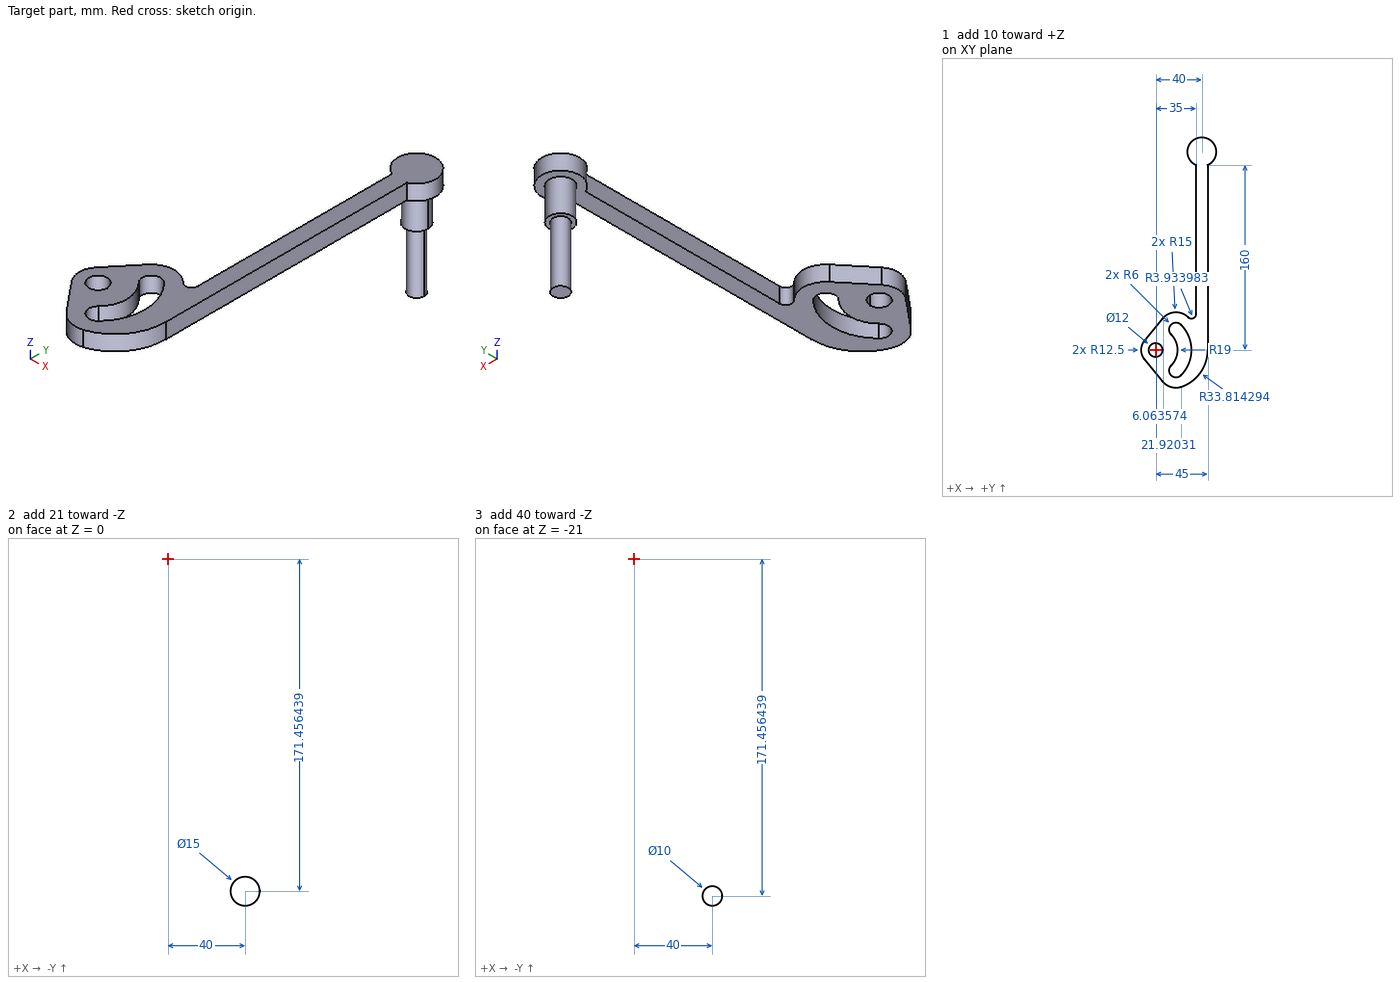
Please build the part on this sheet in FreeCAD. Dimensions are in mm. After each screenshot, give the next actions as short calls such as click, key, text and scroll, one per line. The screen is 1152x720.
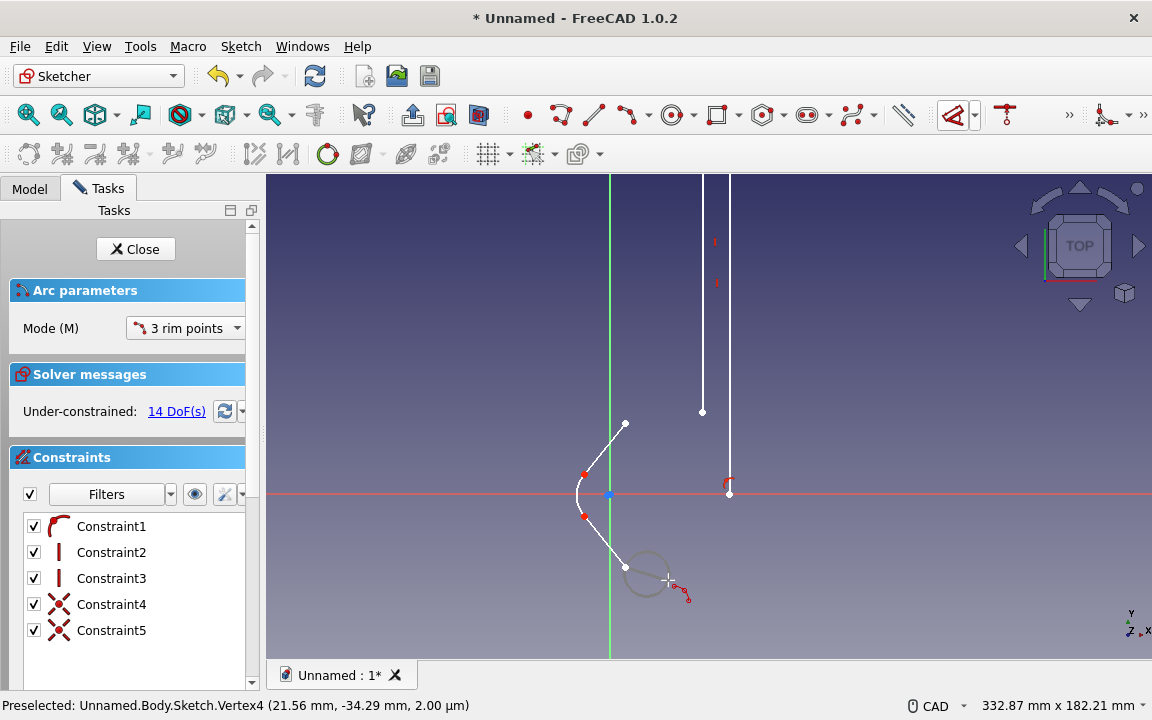
scroll(645, 580, up, 5)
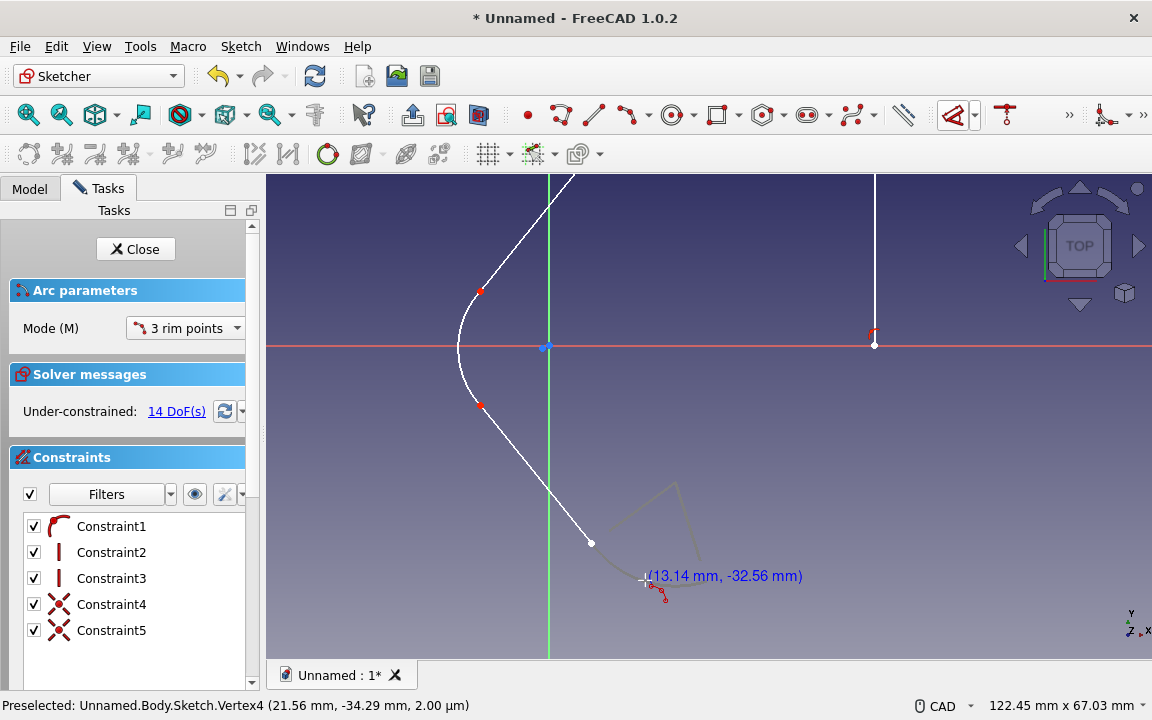
click(645, 577)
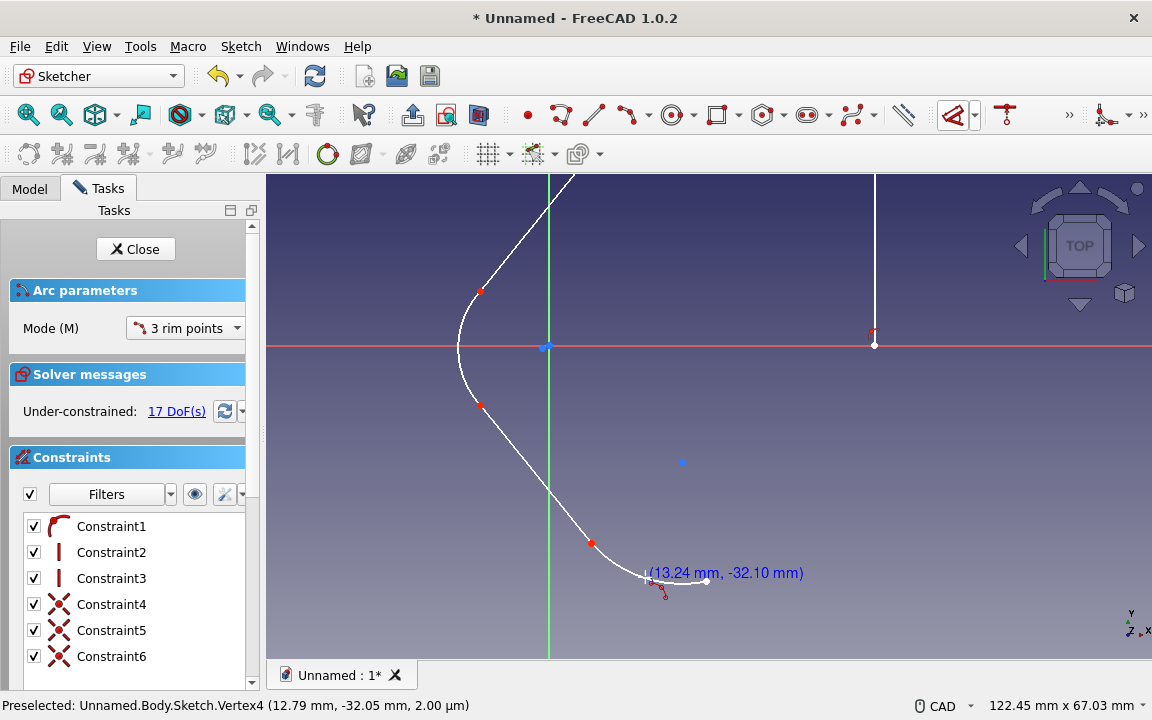
scroll(634, 573, down, 8)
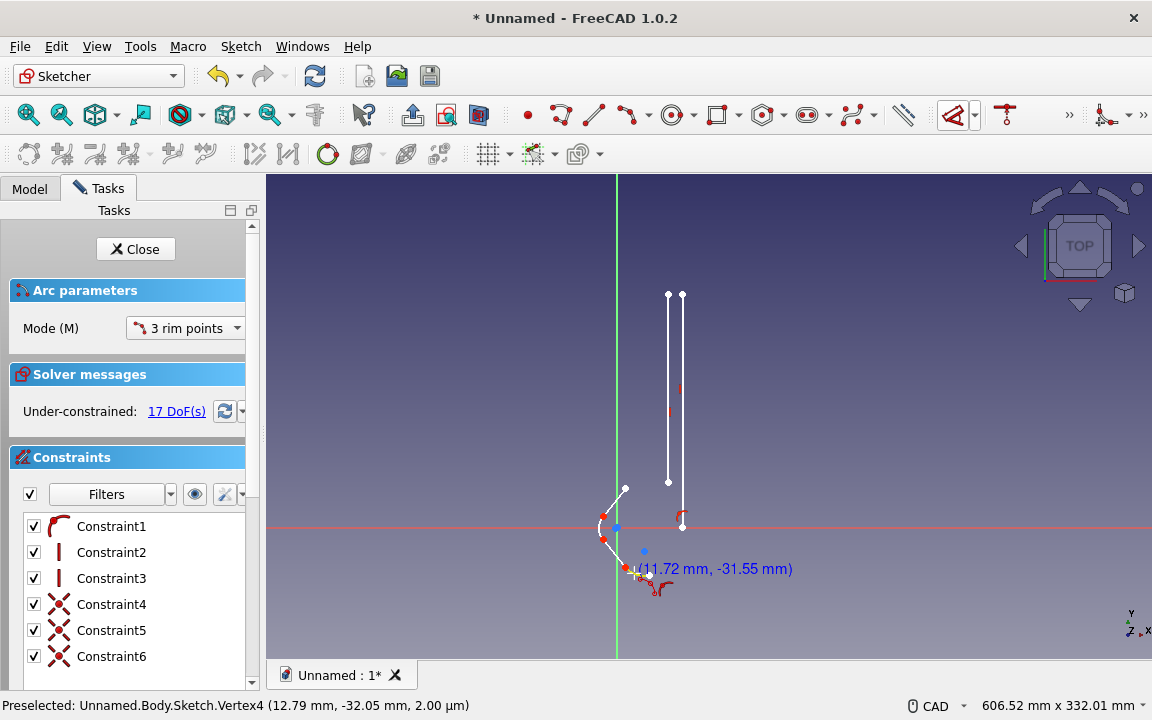
click(649, 575)
click(683, 528)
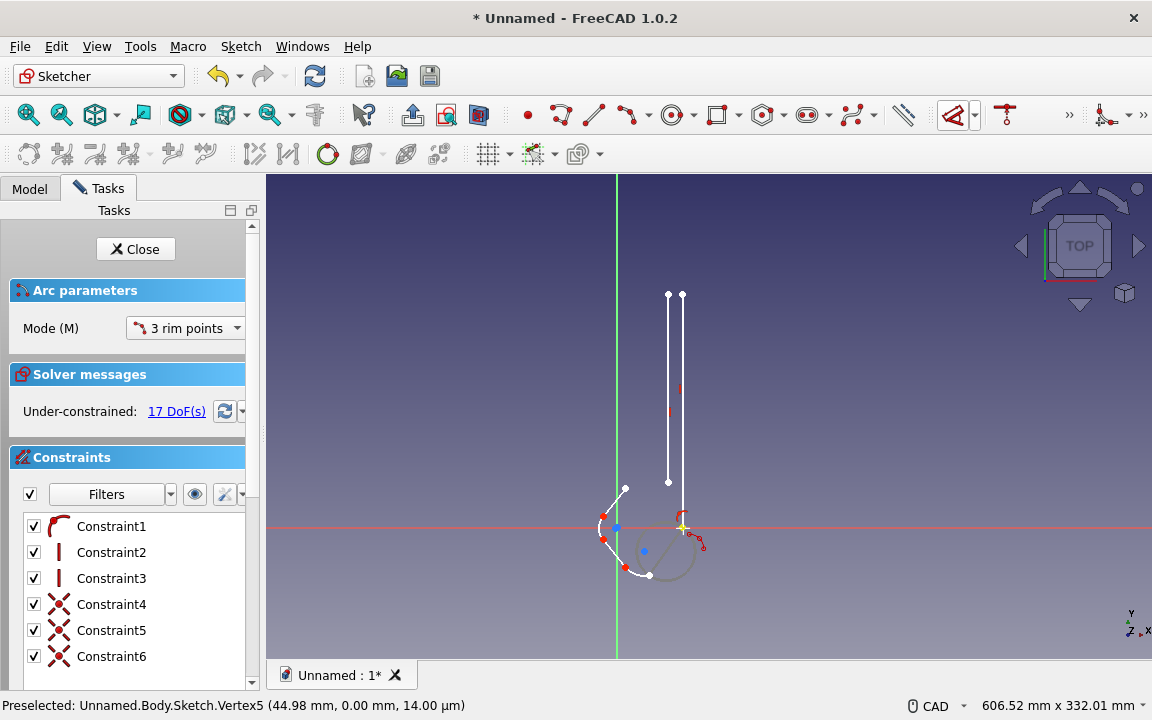
scroll(674, 557, up, 3)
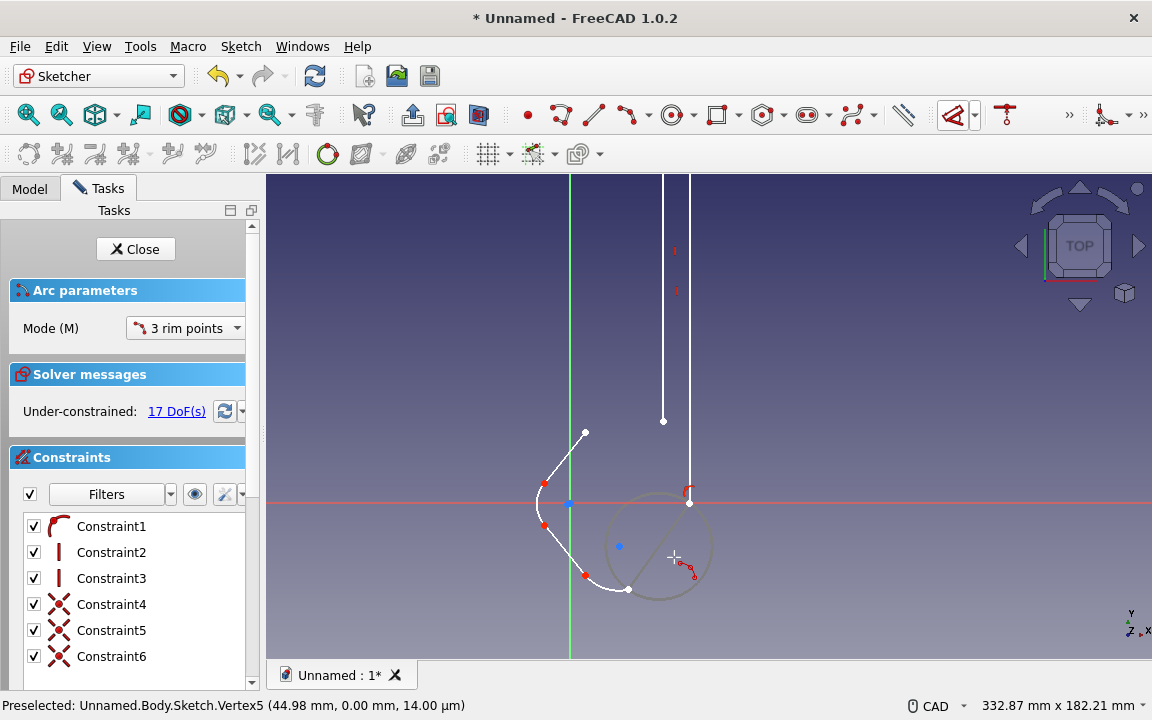
click(673, 556)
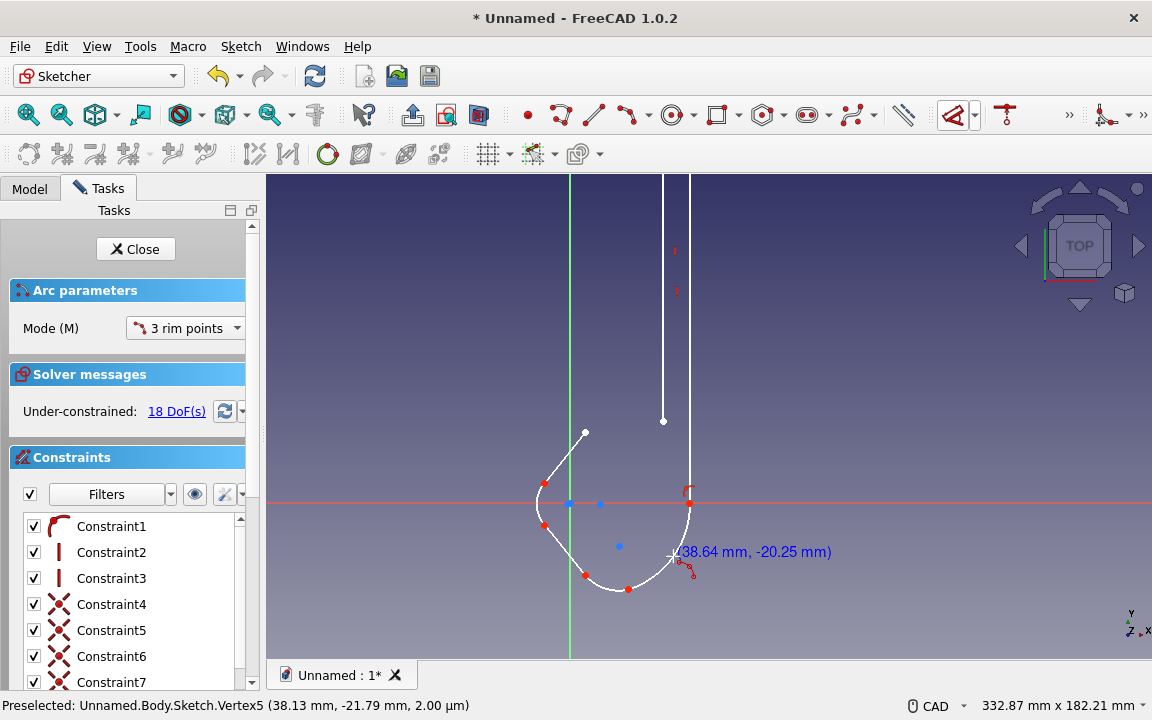
scroll(673, 557, down, 3)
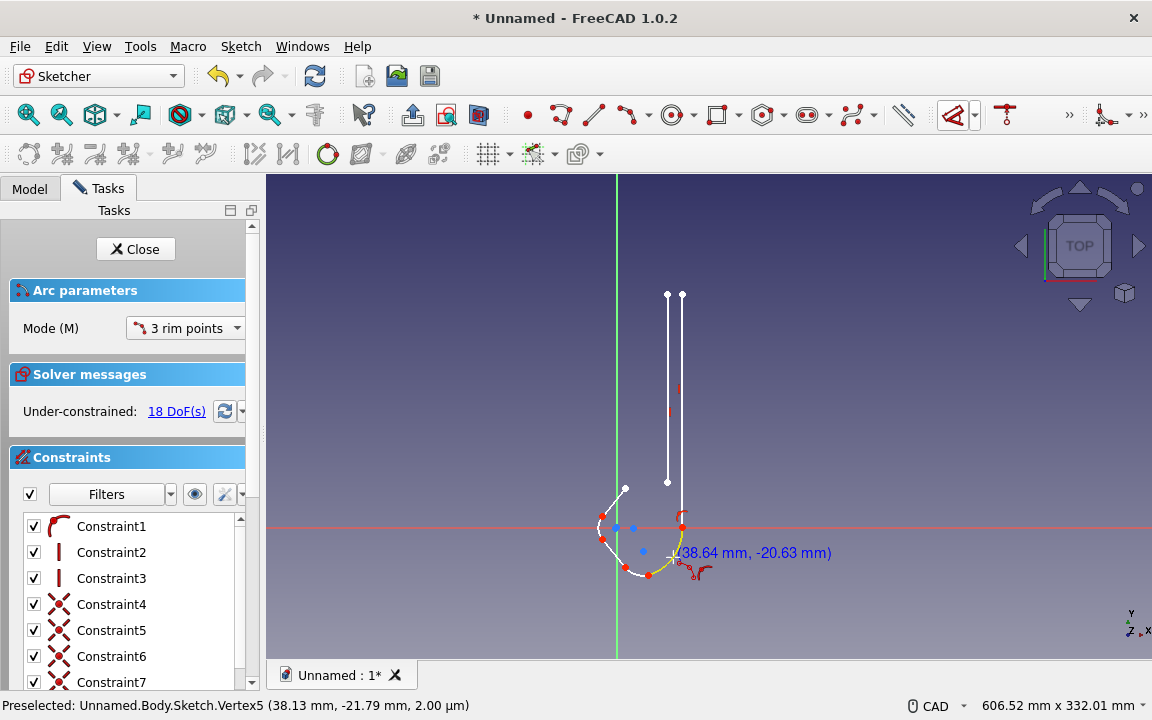
click(682, 295)
click(668, 295)
click(675, 259)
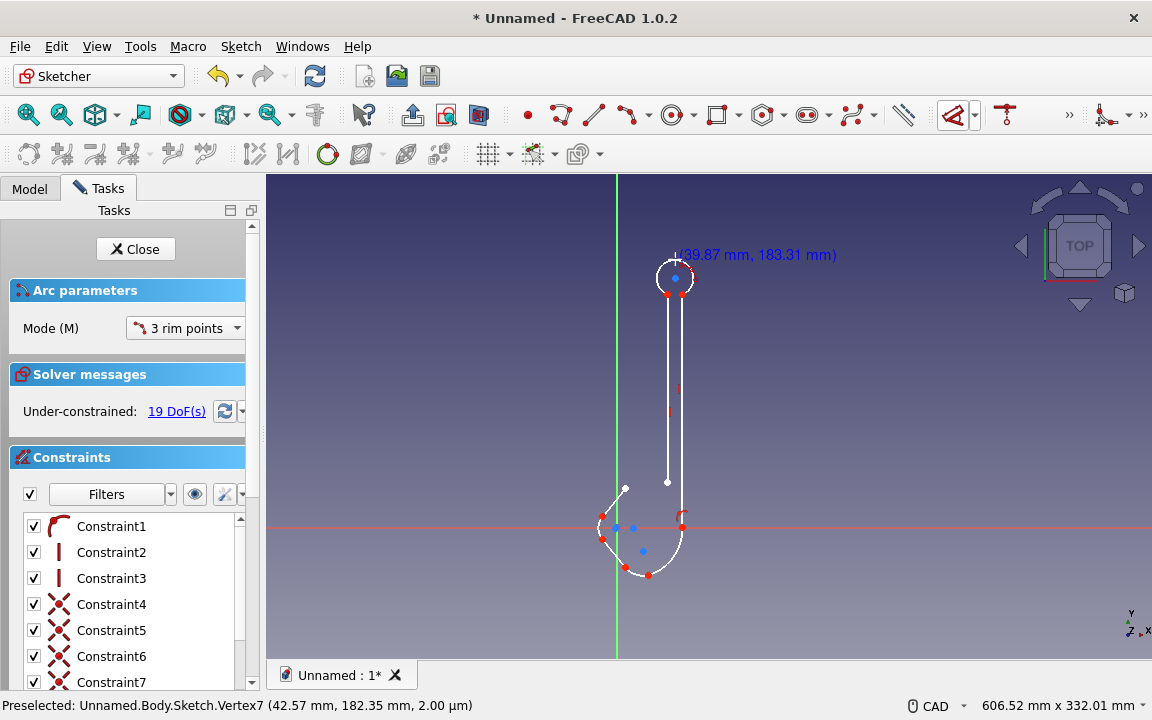
click(668, 483)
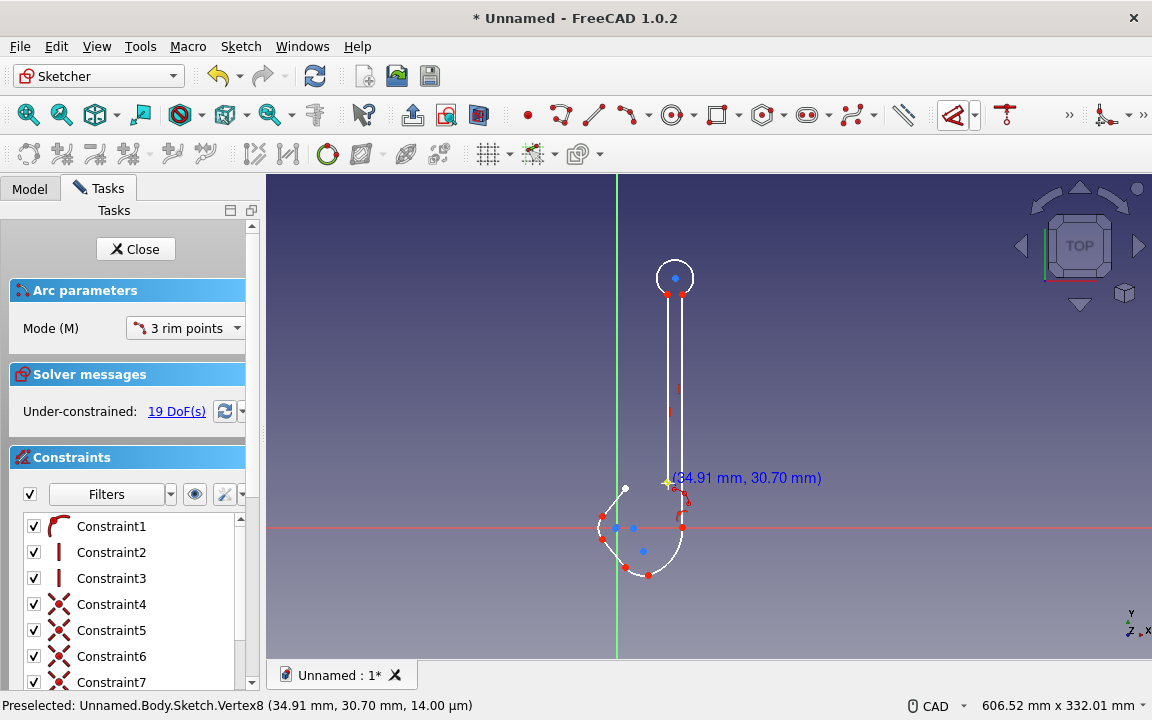
scroll(658, 486, up, 3)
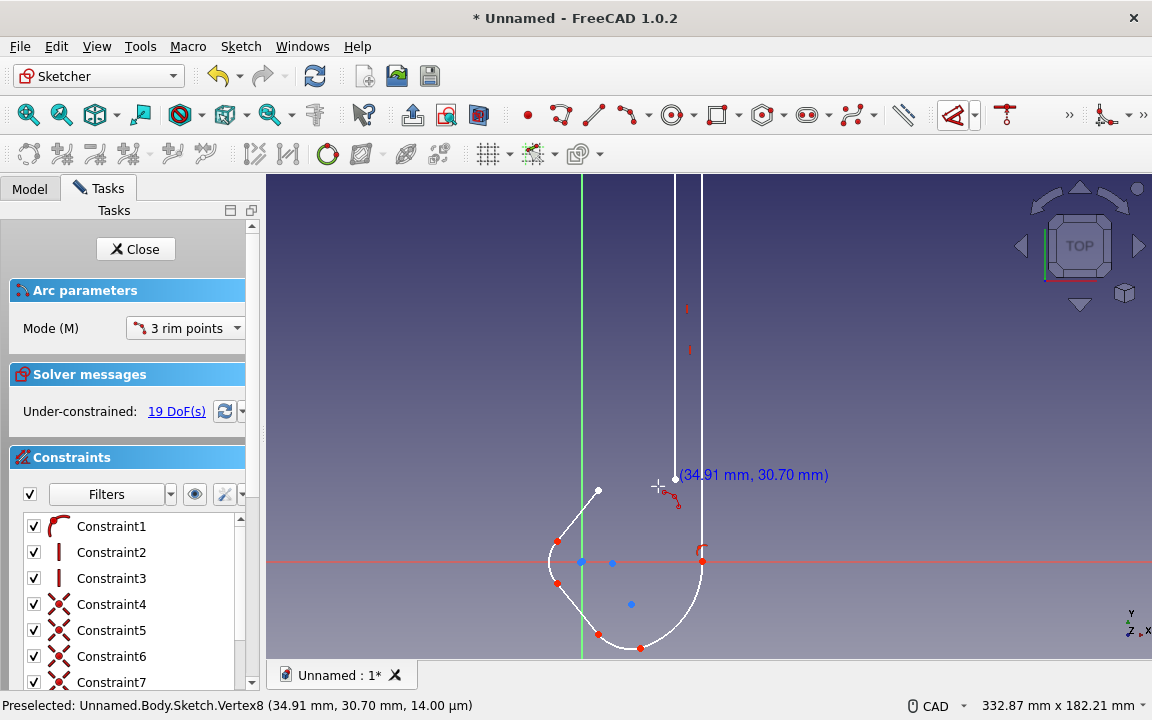
click(658, 486)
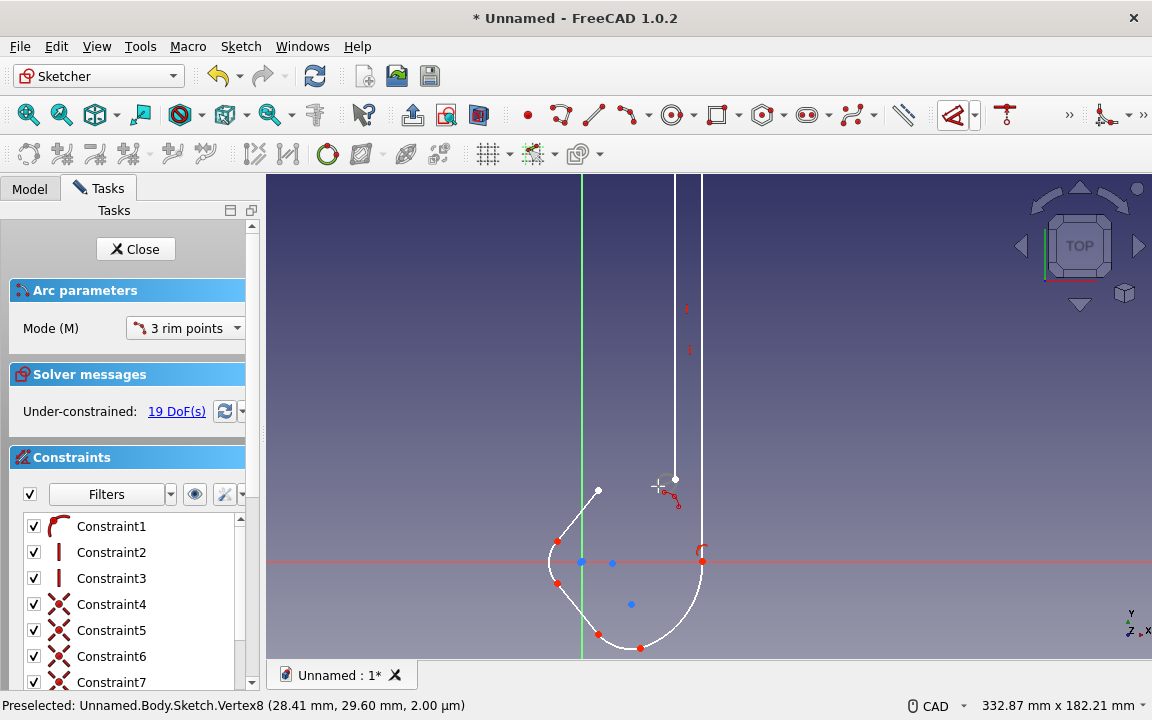
scroll(669, 489, up, 5)